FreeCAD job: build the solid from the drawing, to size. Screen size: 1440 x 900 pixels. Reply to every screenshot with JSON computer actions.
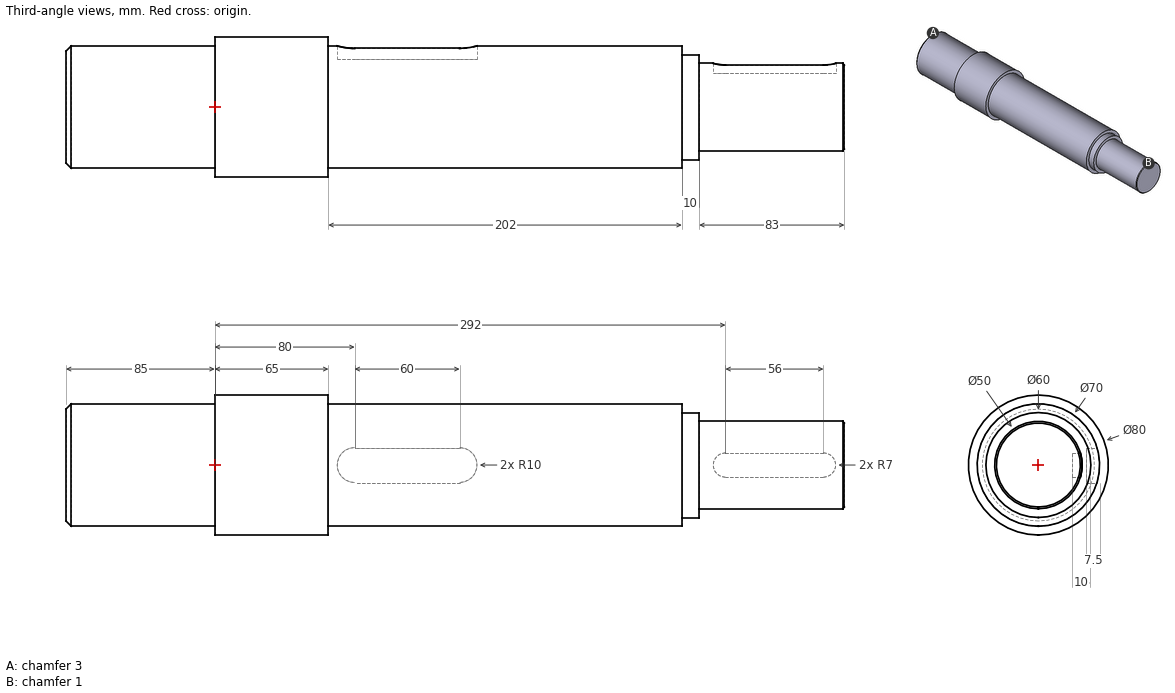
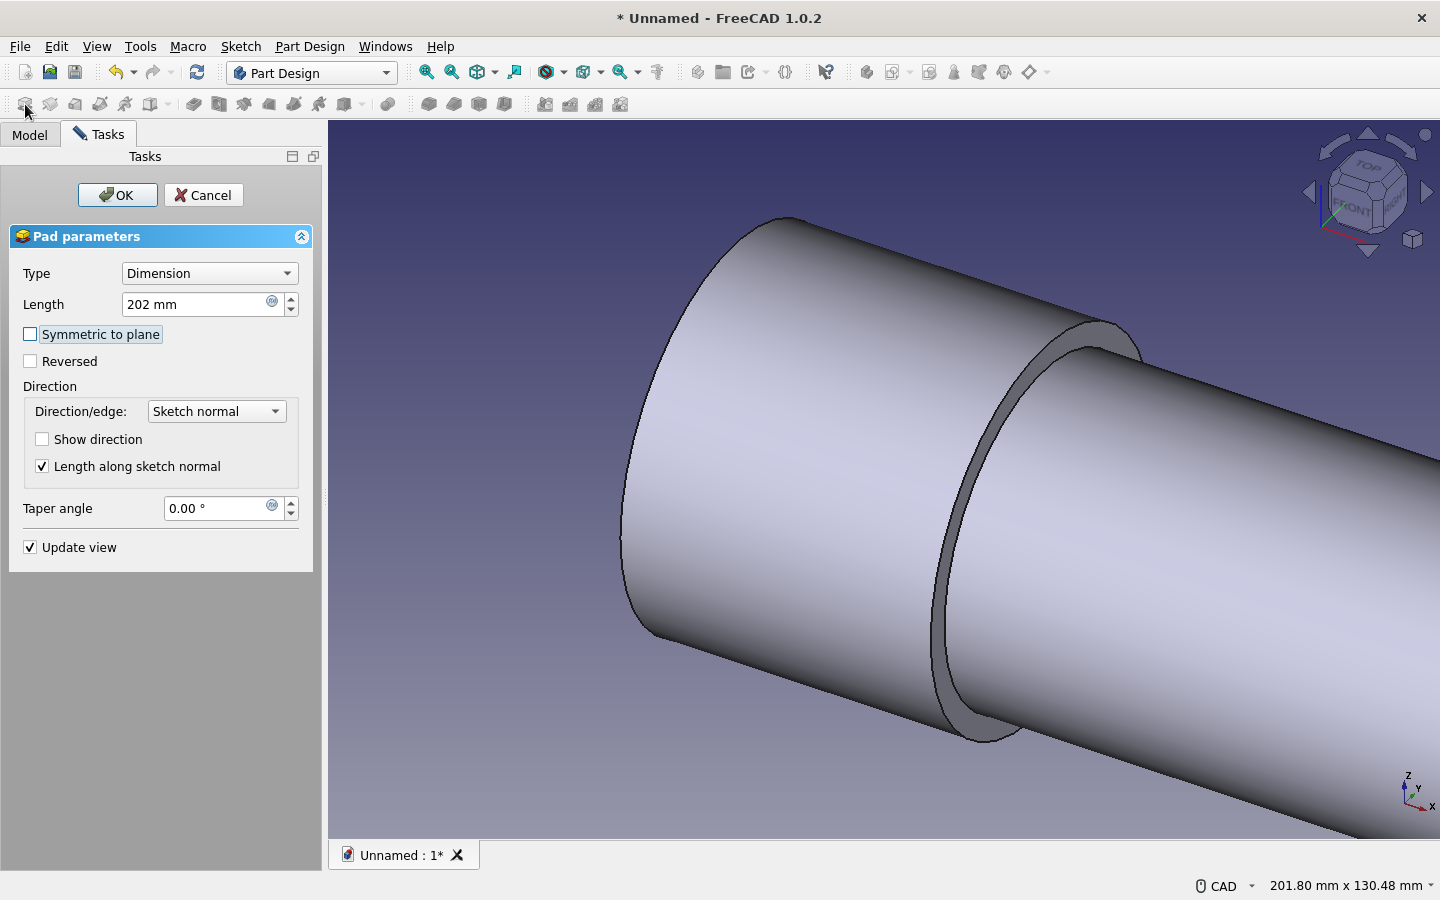
{"action": "left_click", "coordinate": [118, 195]}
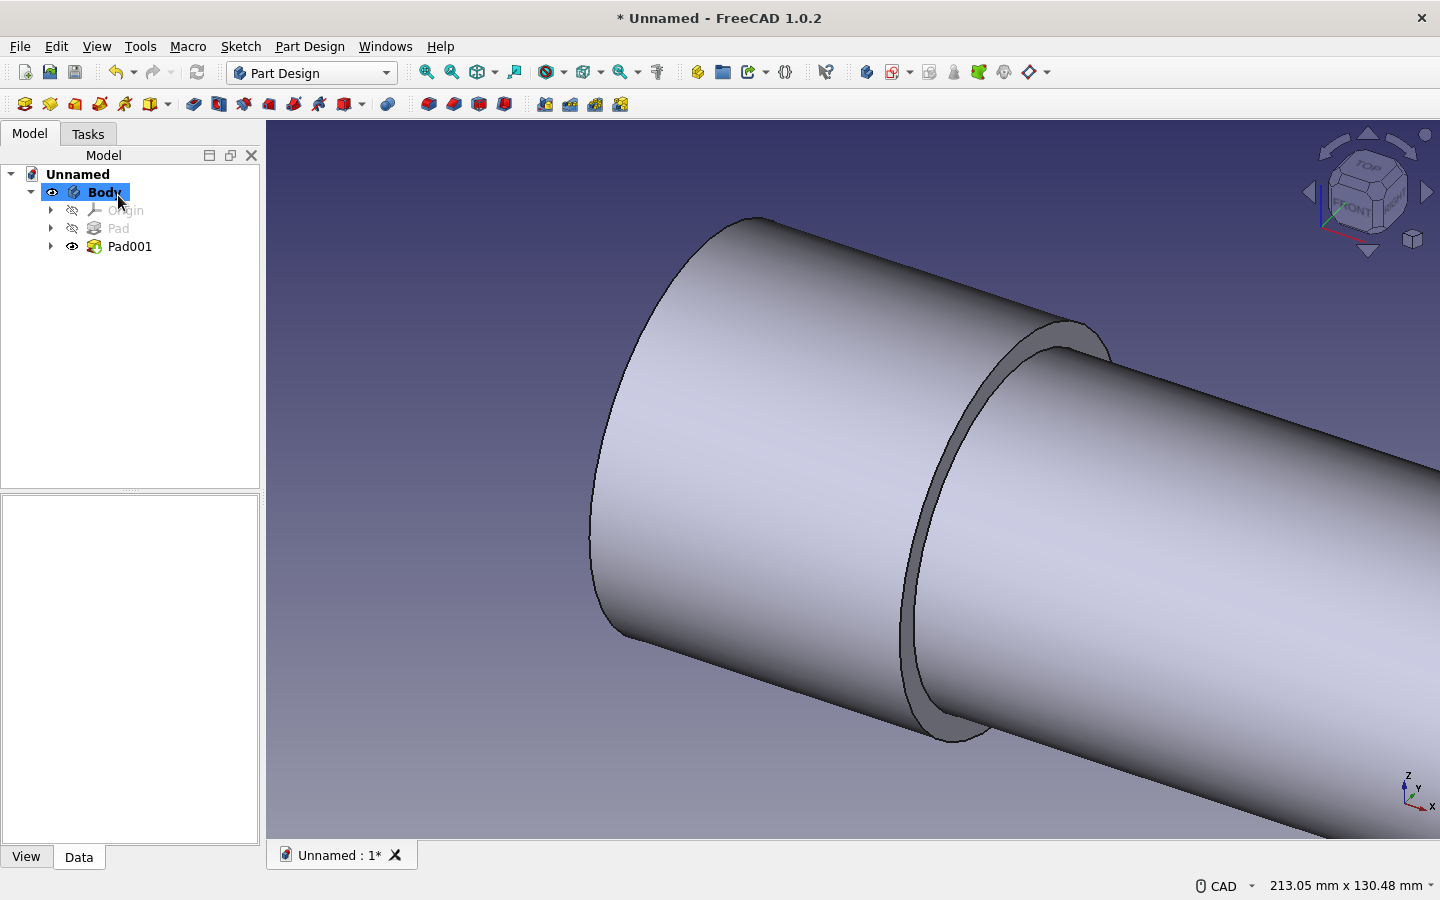
{"action": "key", "text": "v f"}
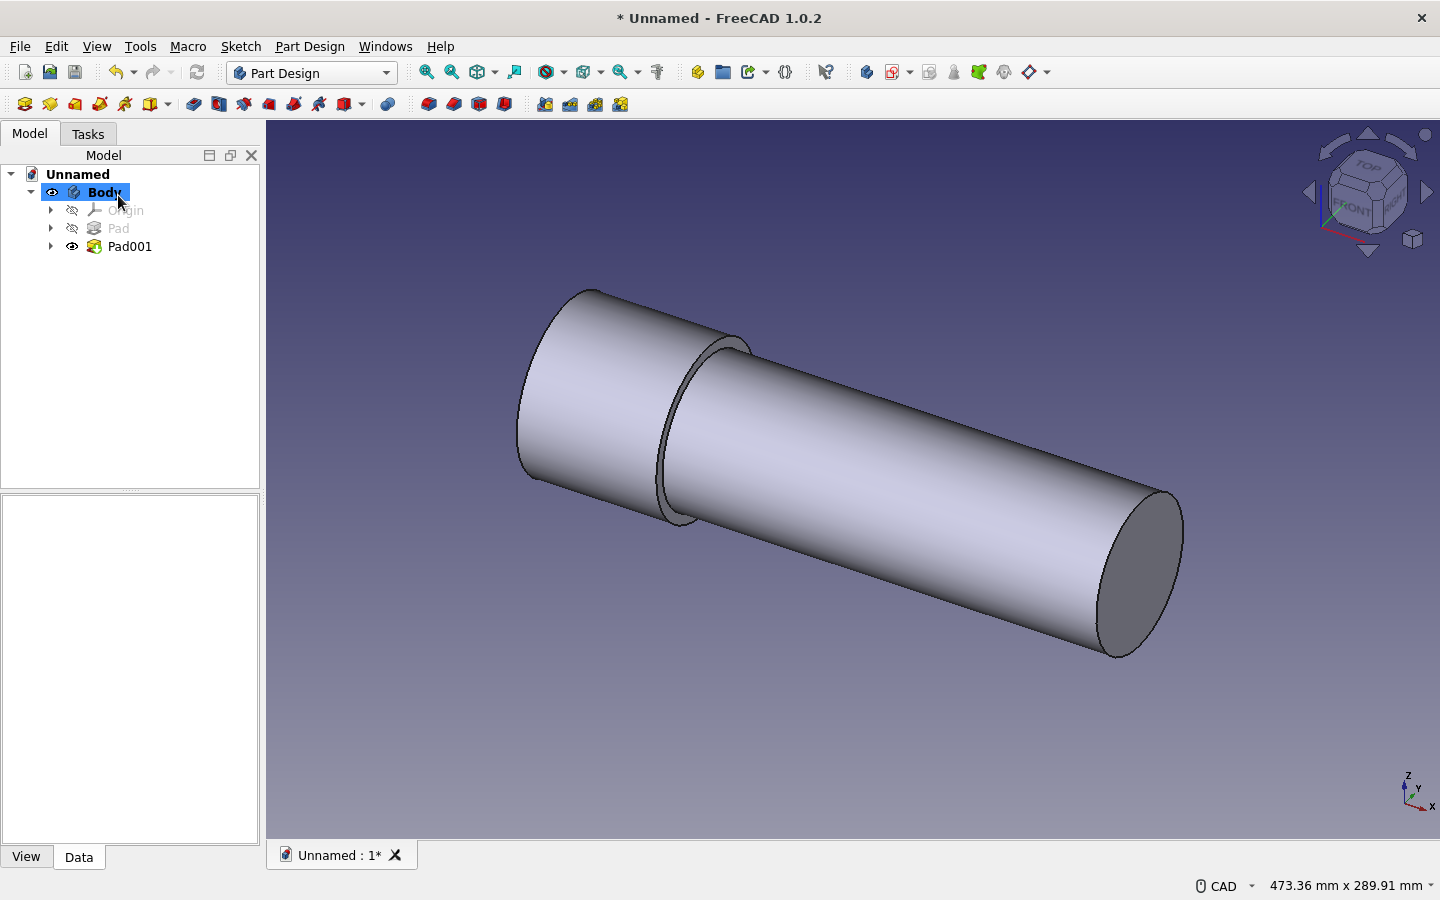
{"action": "left_click", "coordinate": [51, 210]}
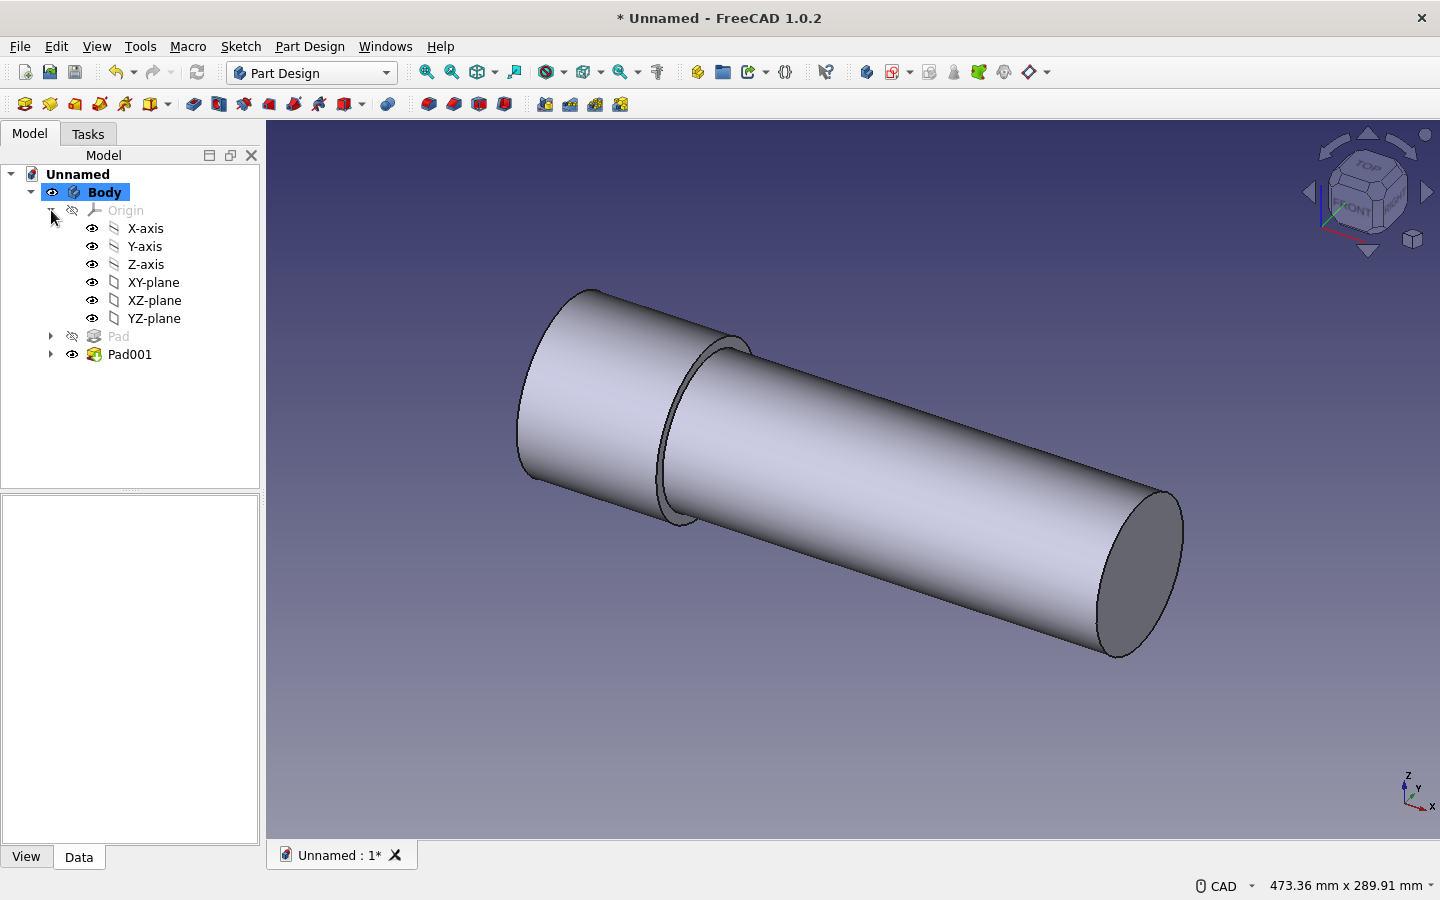
{"action": "left_click", "coordinate": [137, 318]}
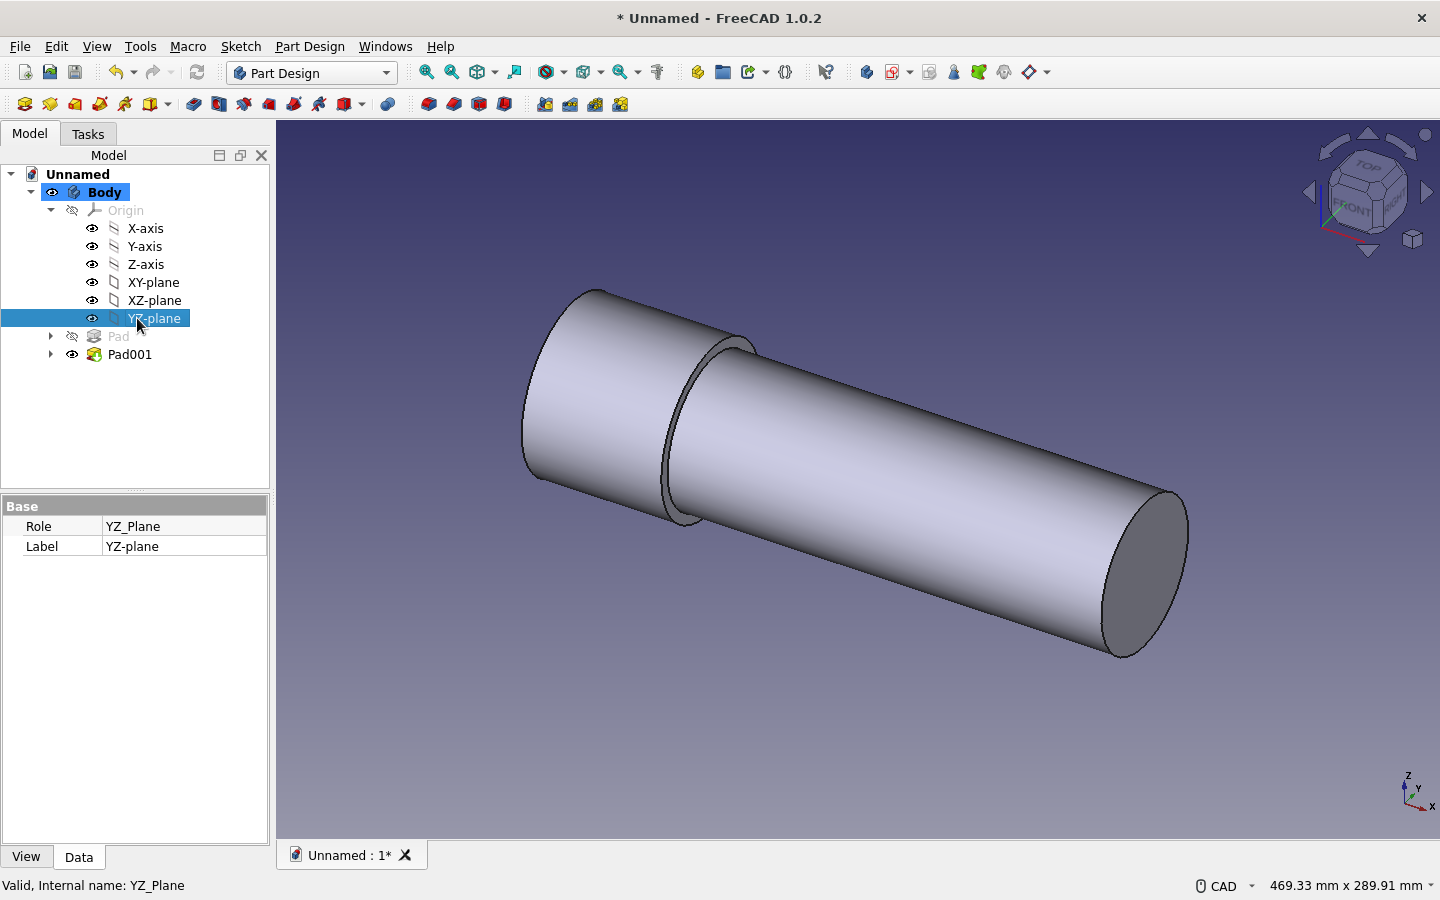
{"action": "left_click", "coordinate": [1028, 72]}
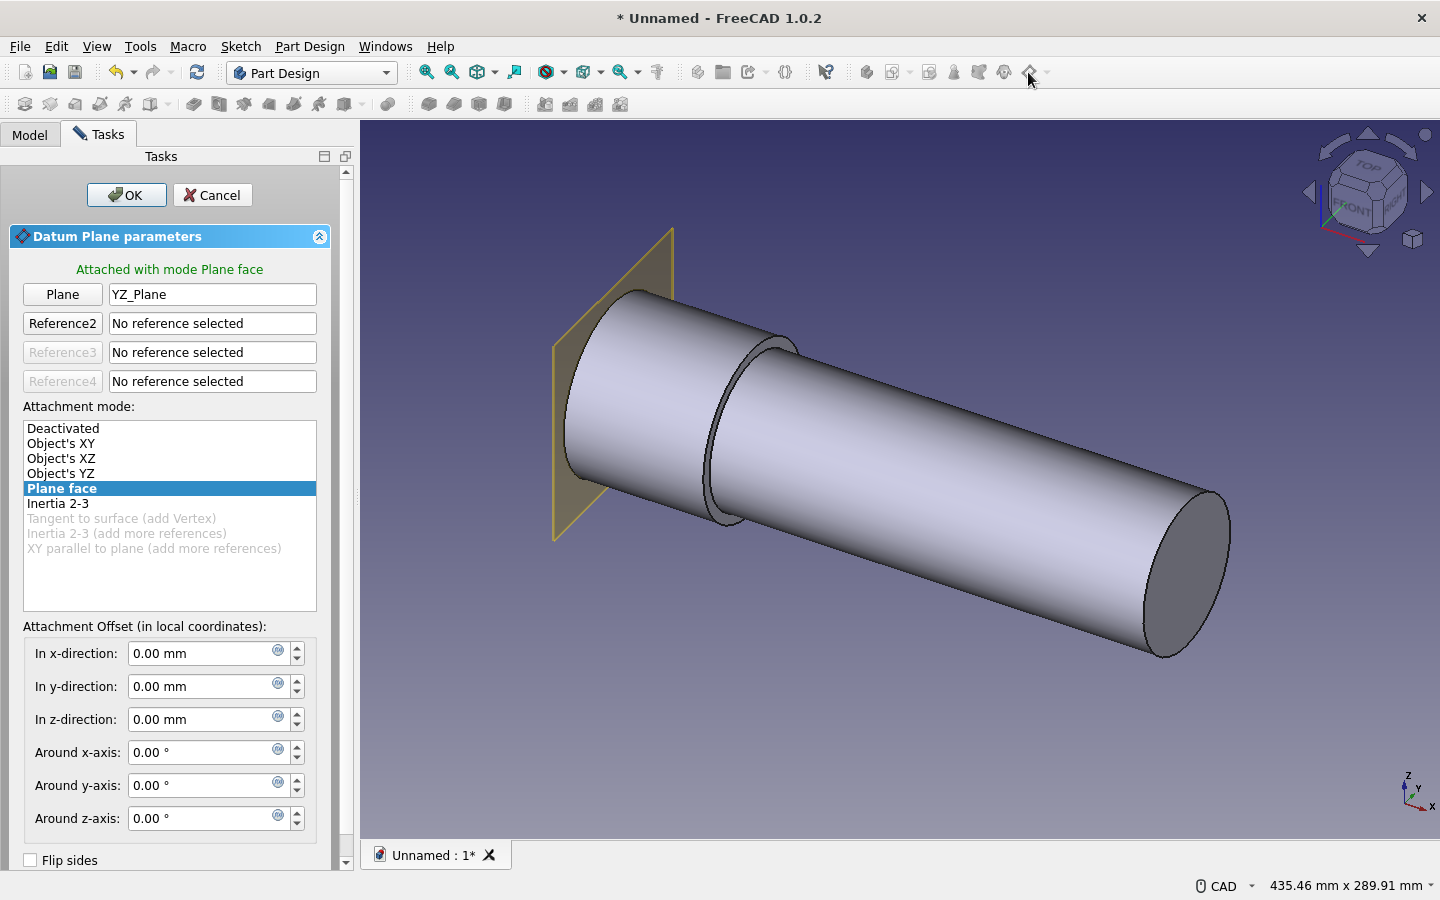
{"action": "triple_click", "coordinate": [210, 720]}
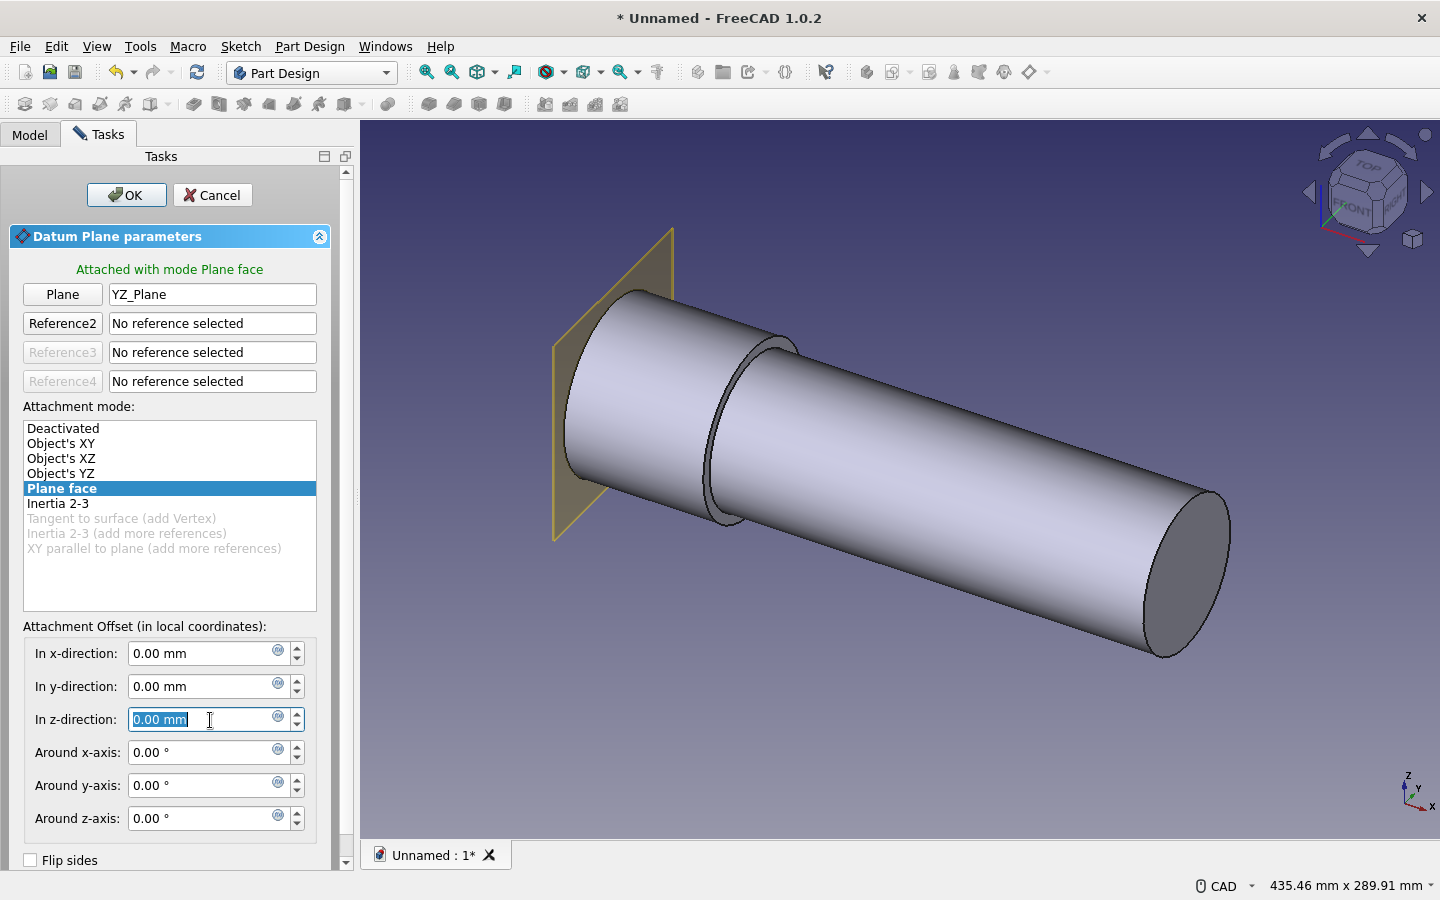
{"action": "type", "text": "-85"}
{"action": "key", "text": "Tab"}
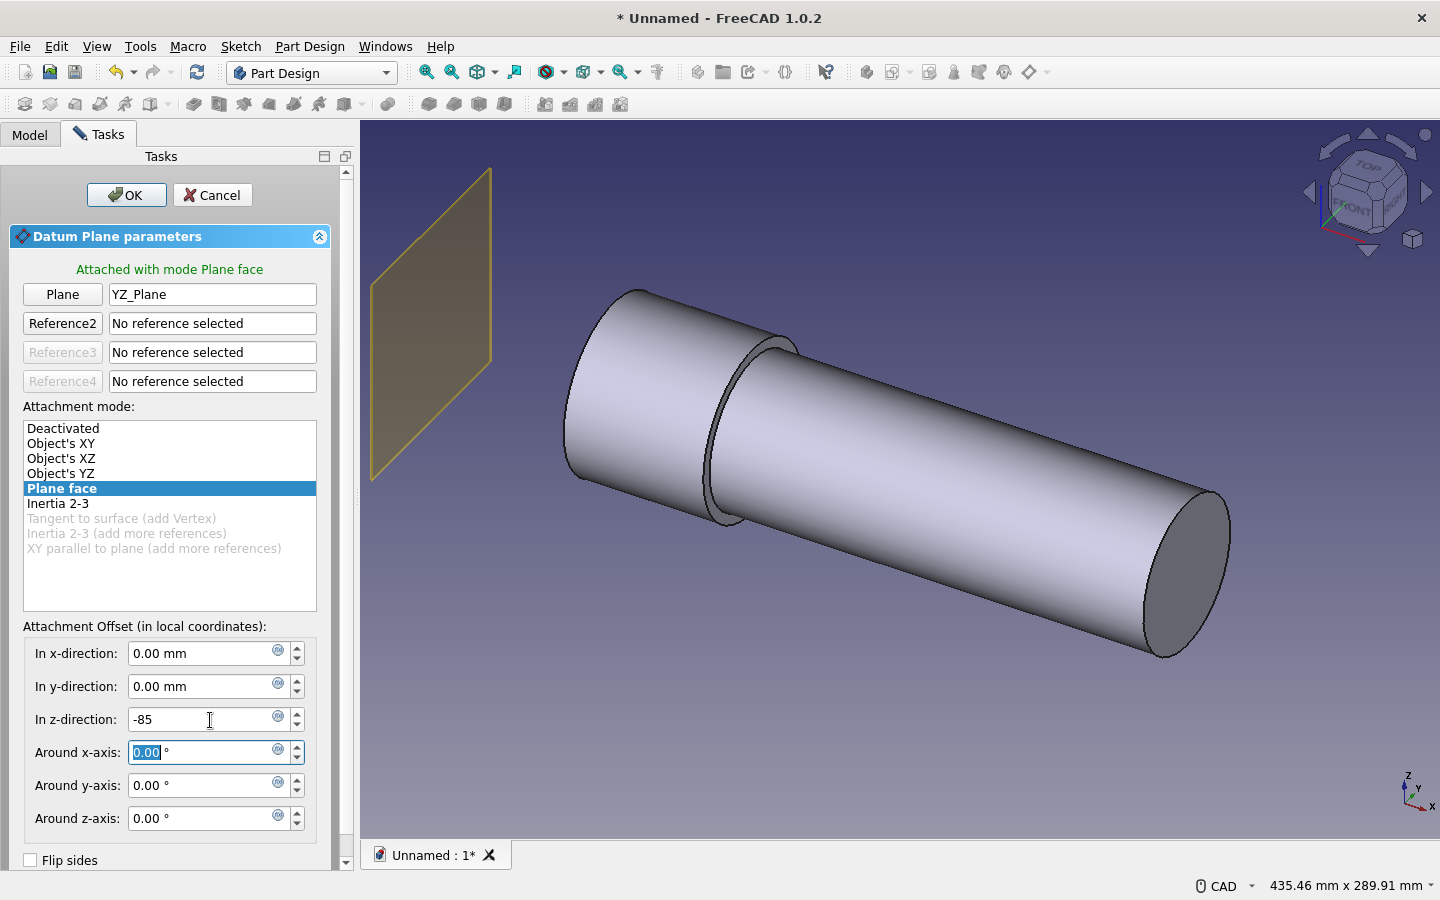
{"action": "left_click", "coordinate": [127, 195]}